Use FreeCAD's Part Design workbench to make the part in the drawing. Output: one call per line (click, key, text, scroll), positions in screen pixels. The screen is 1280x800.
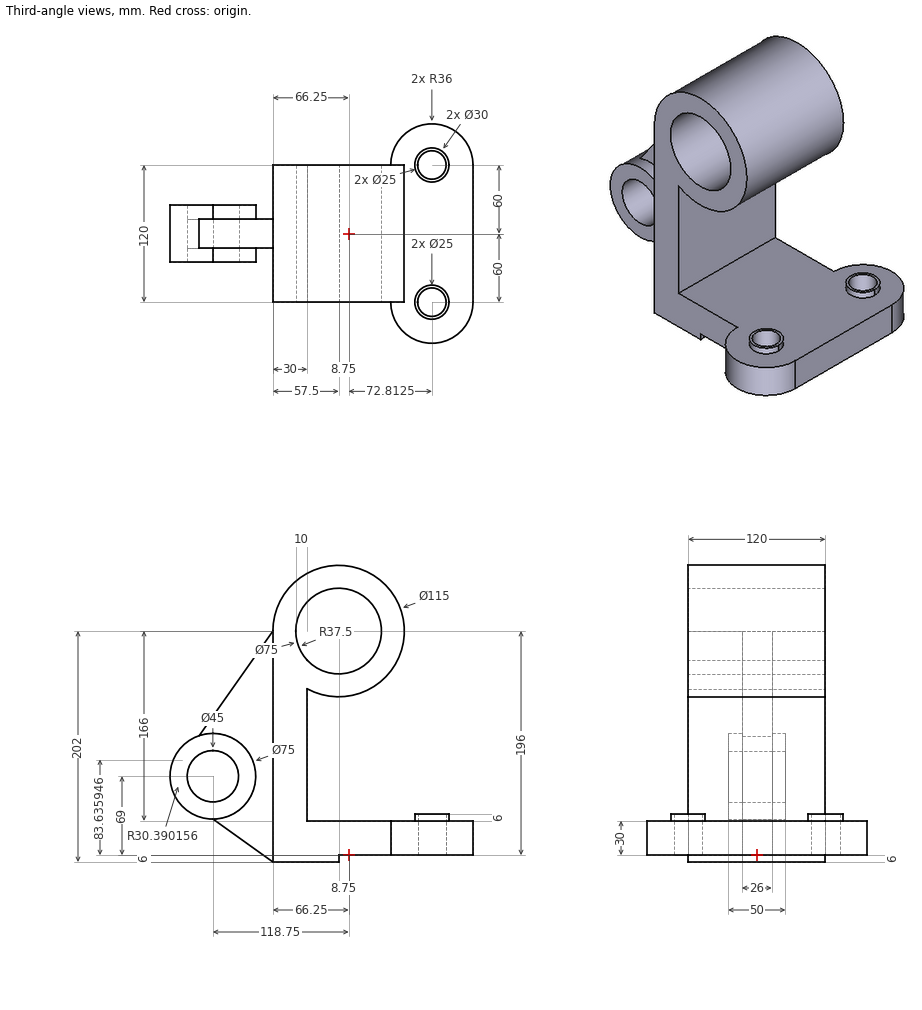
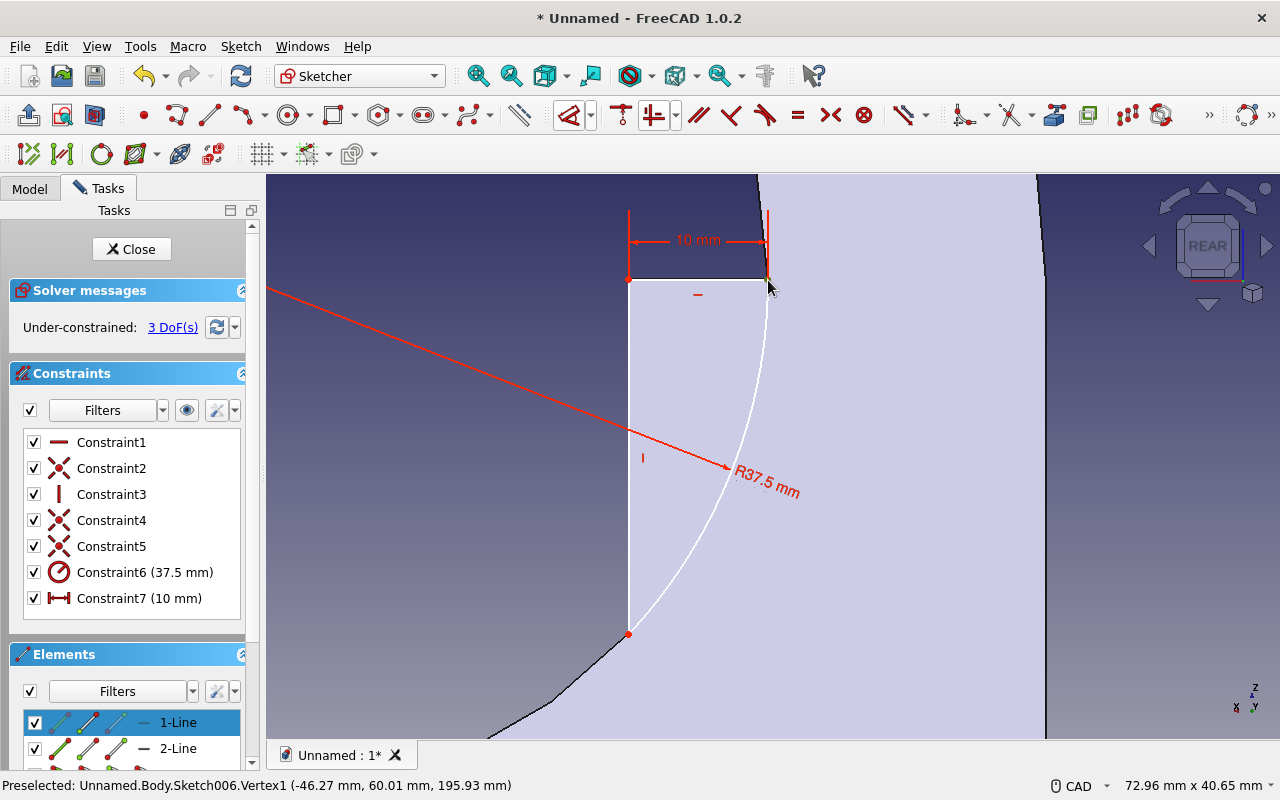
key(i)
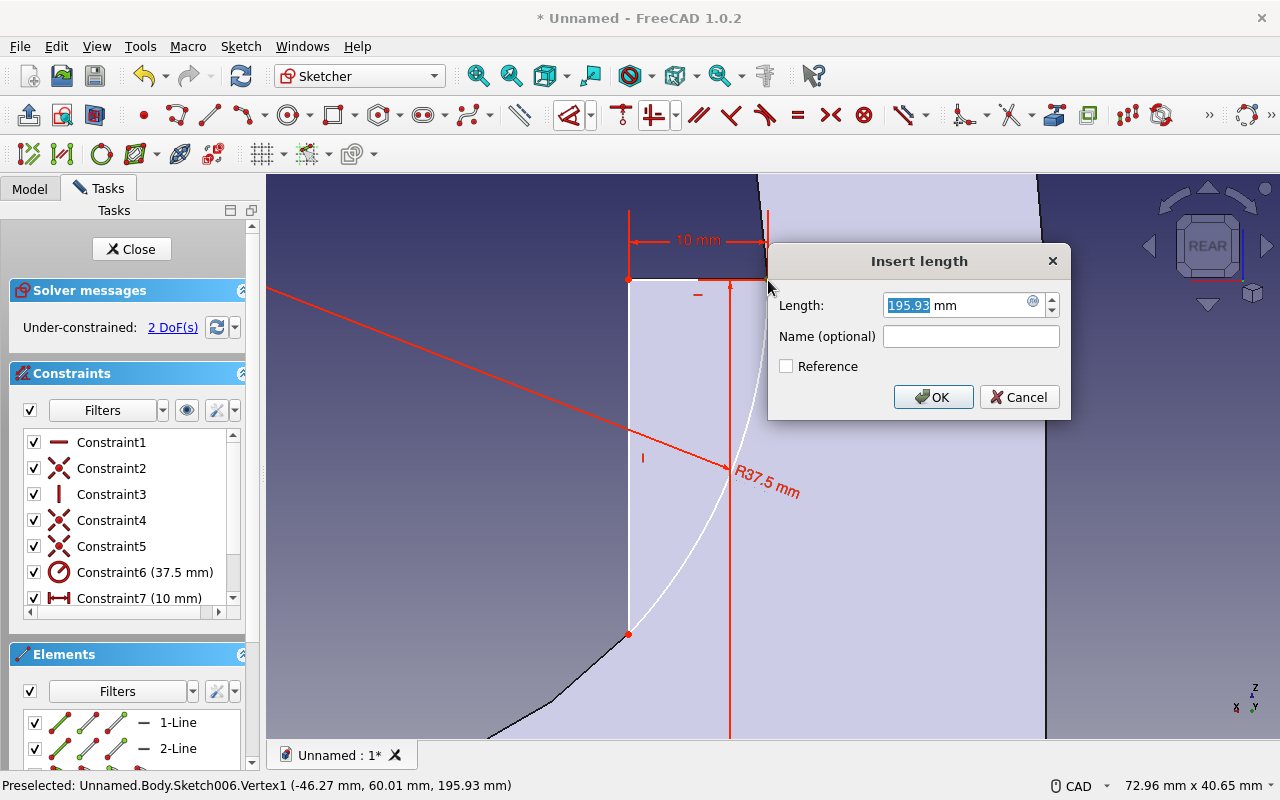
text(196)
key(Return)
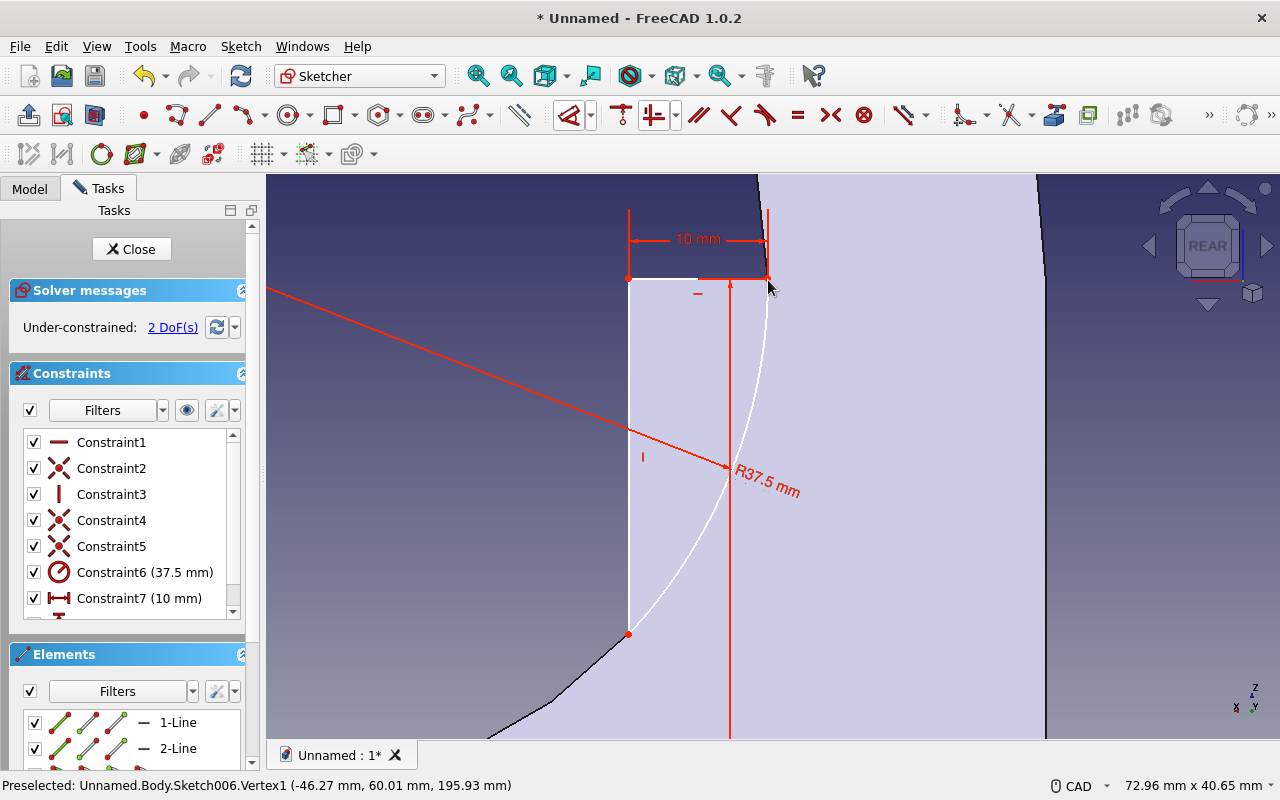
scroll(1115, 458, down, 1)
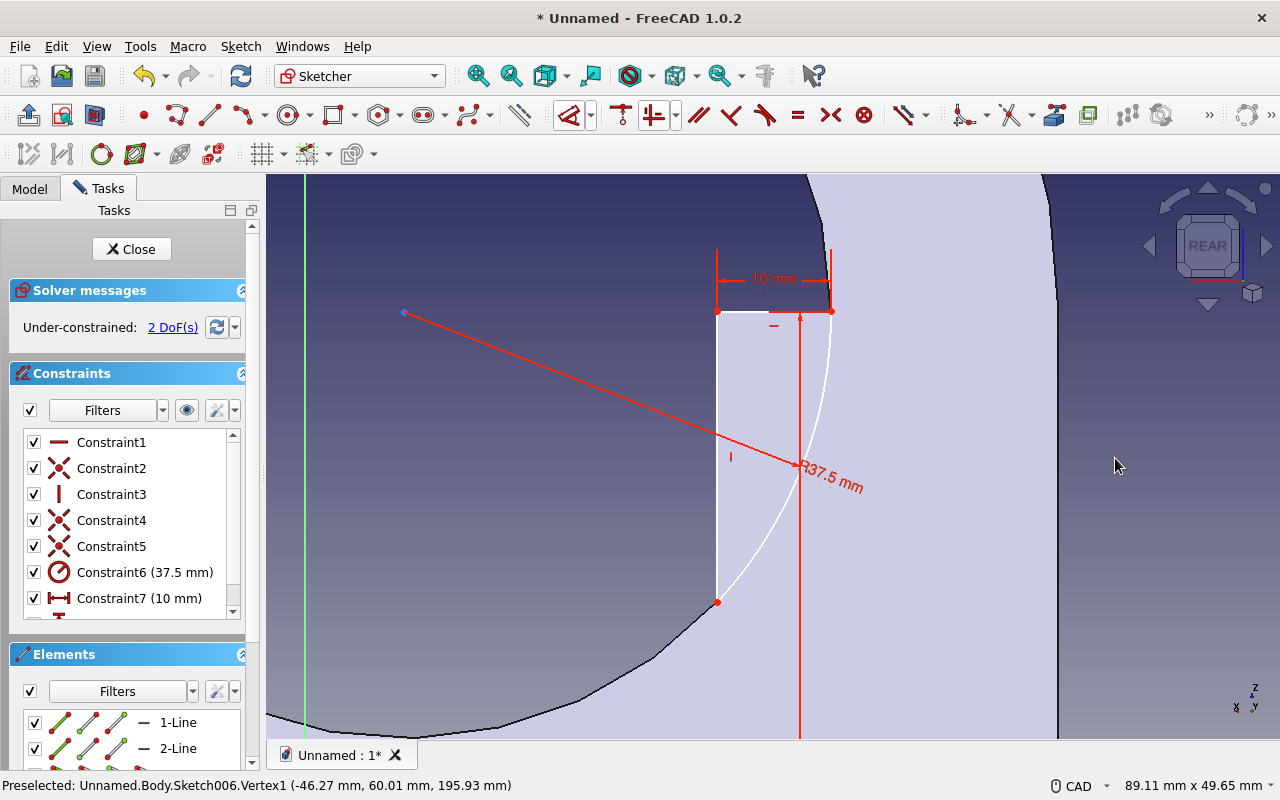
click(404, 312)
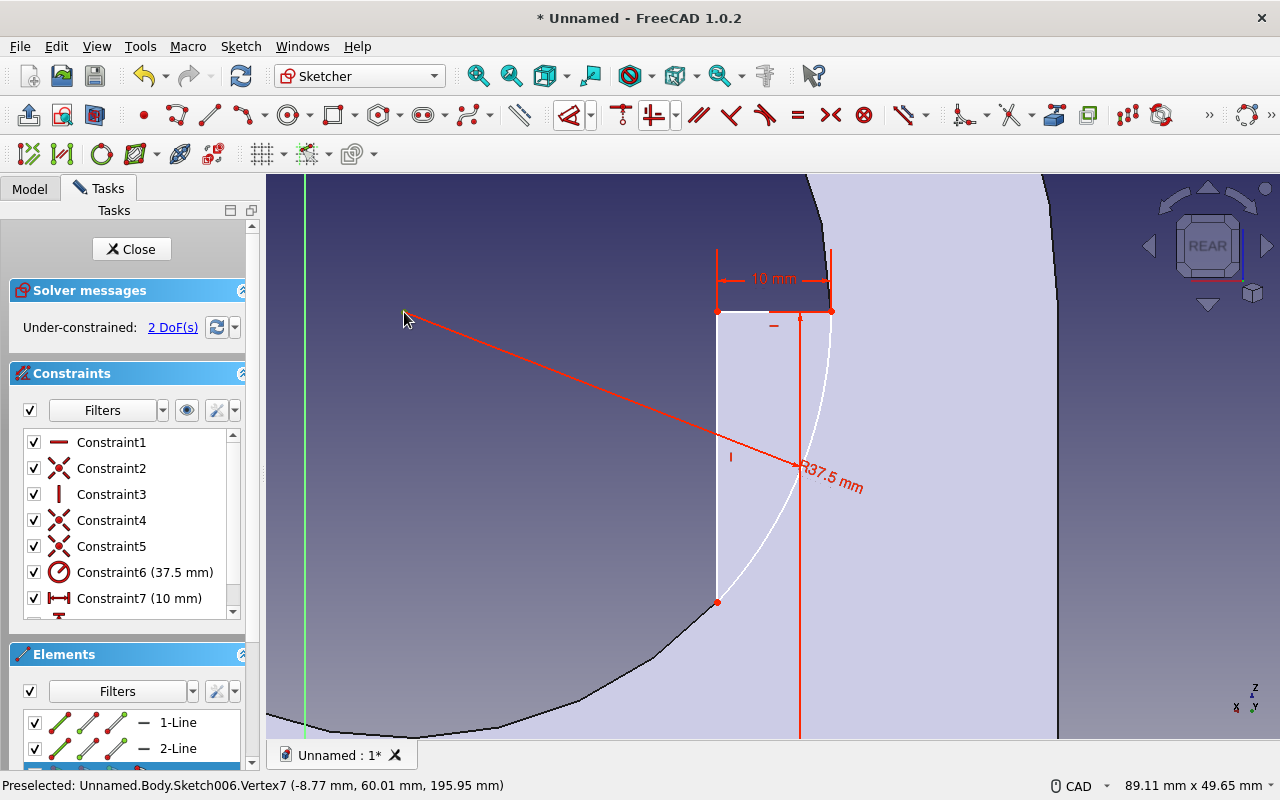
key(i)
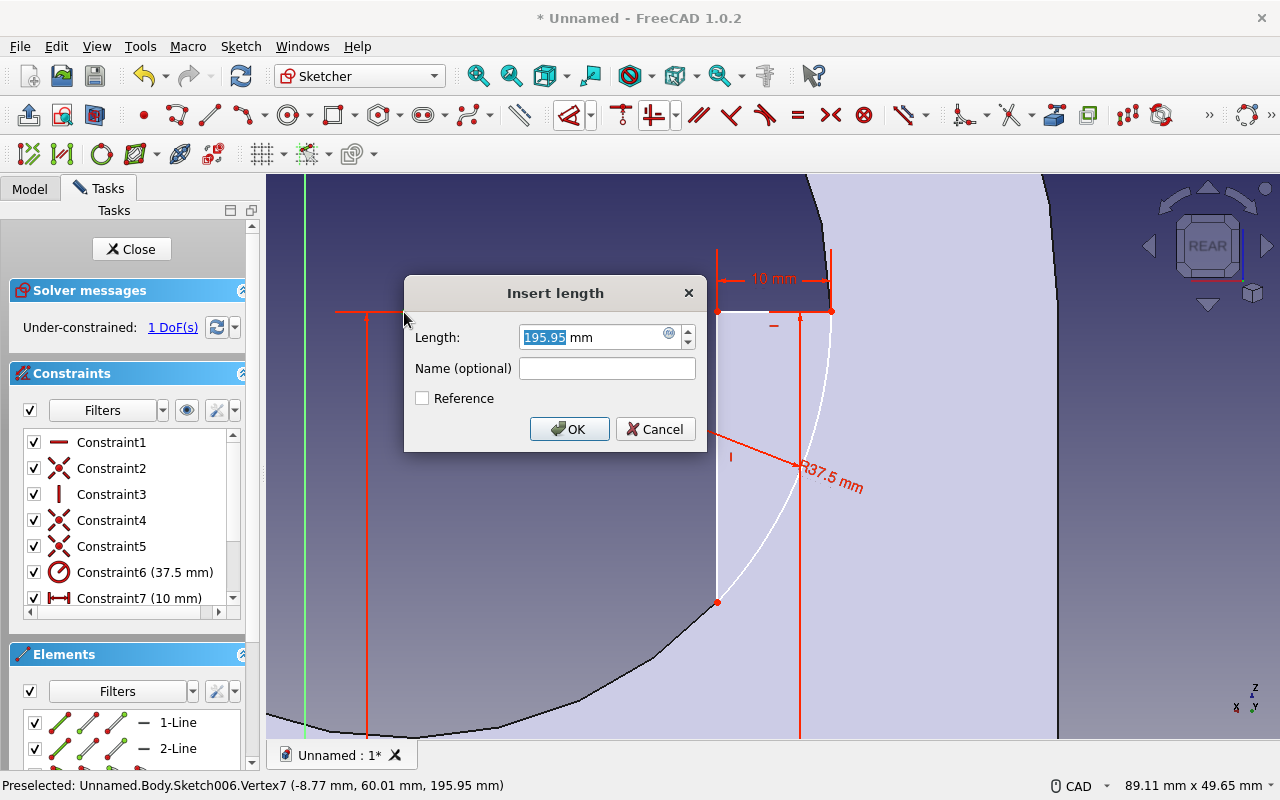
text(196)
key(Return)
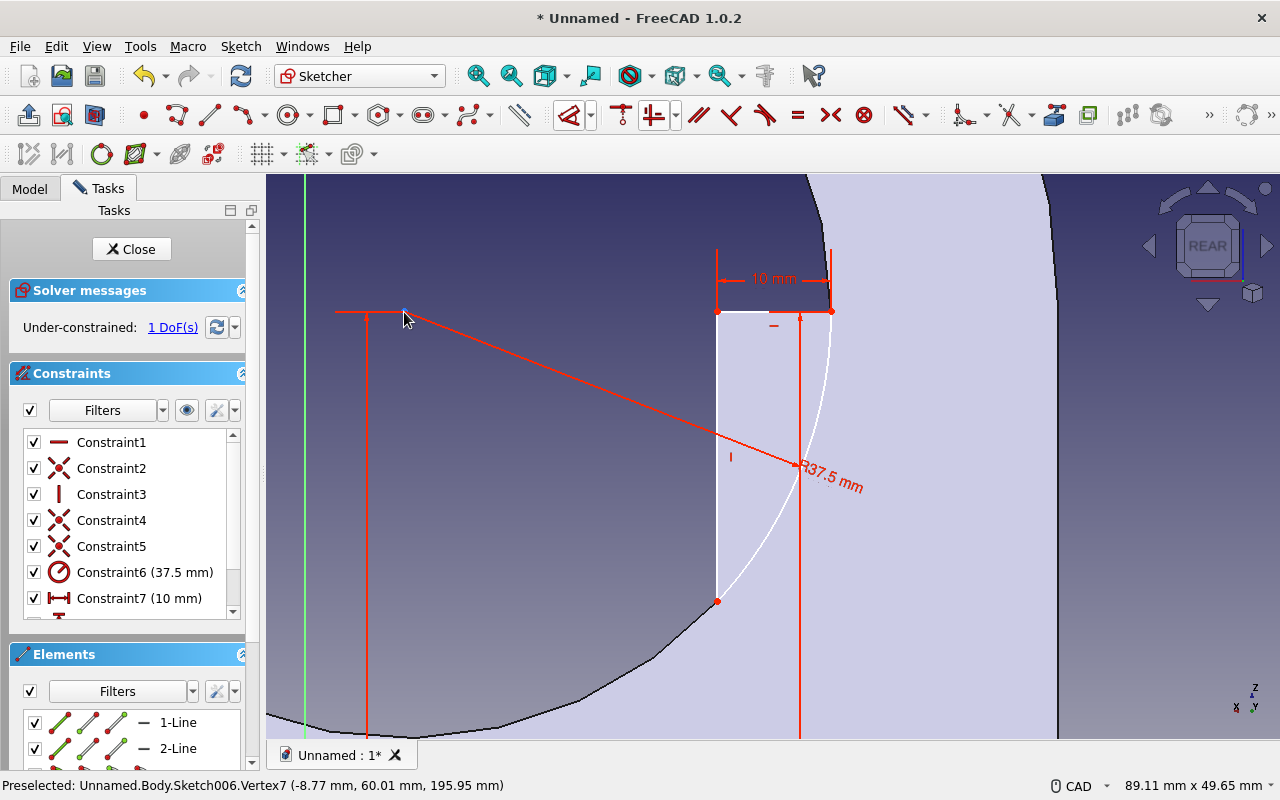
click(404, 312)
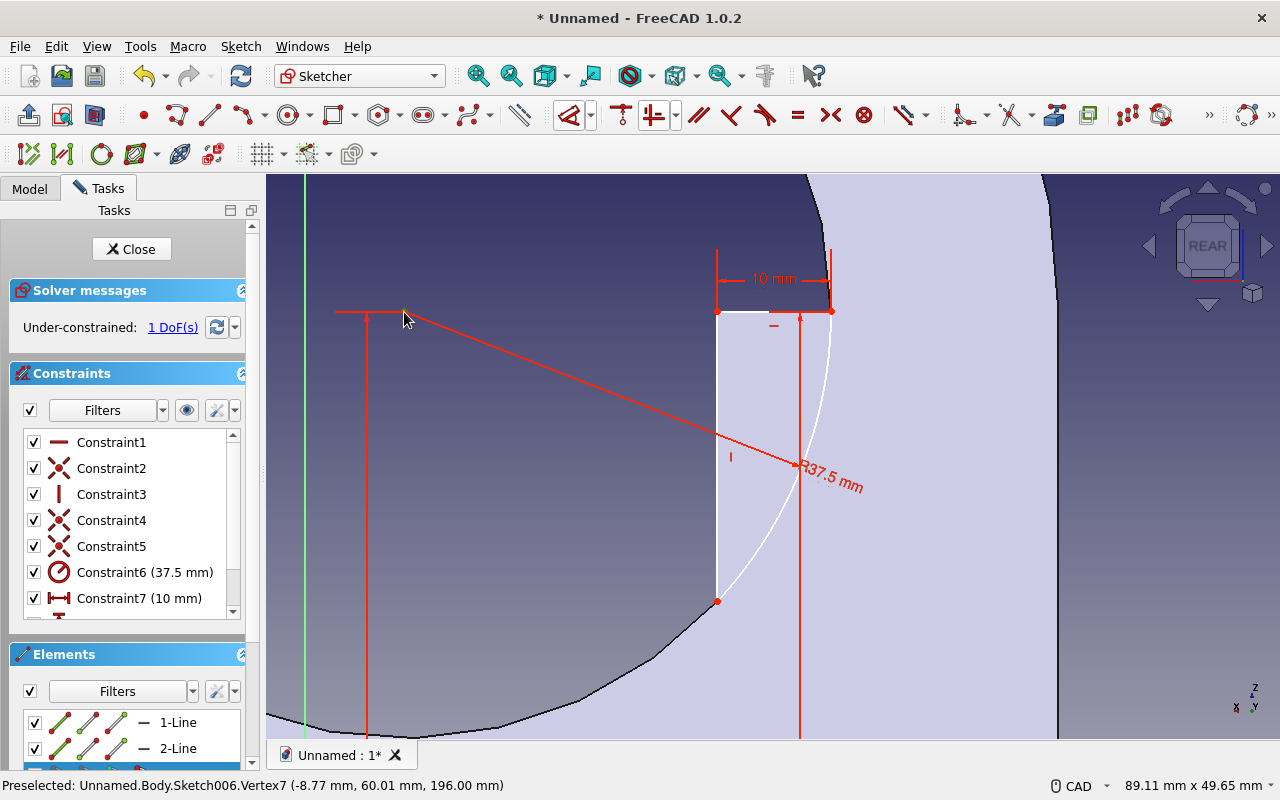
click(590, 116)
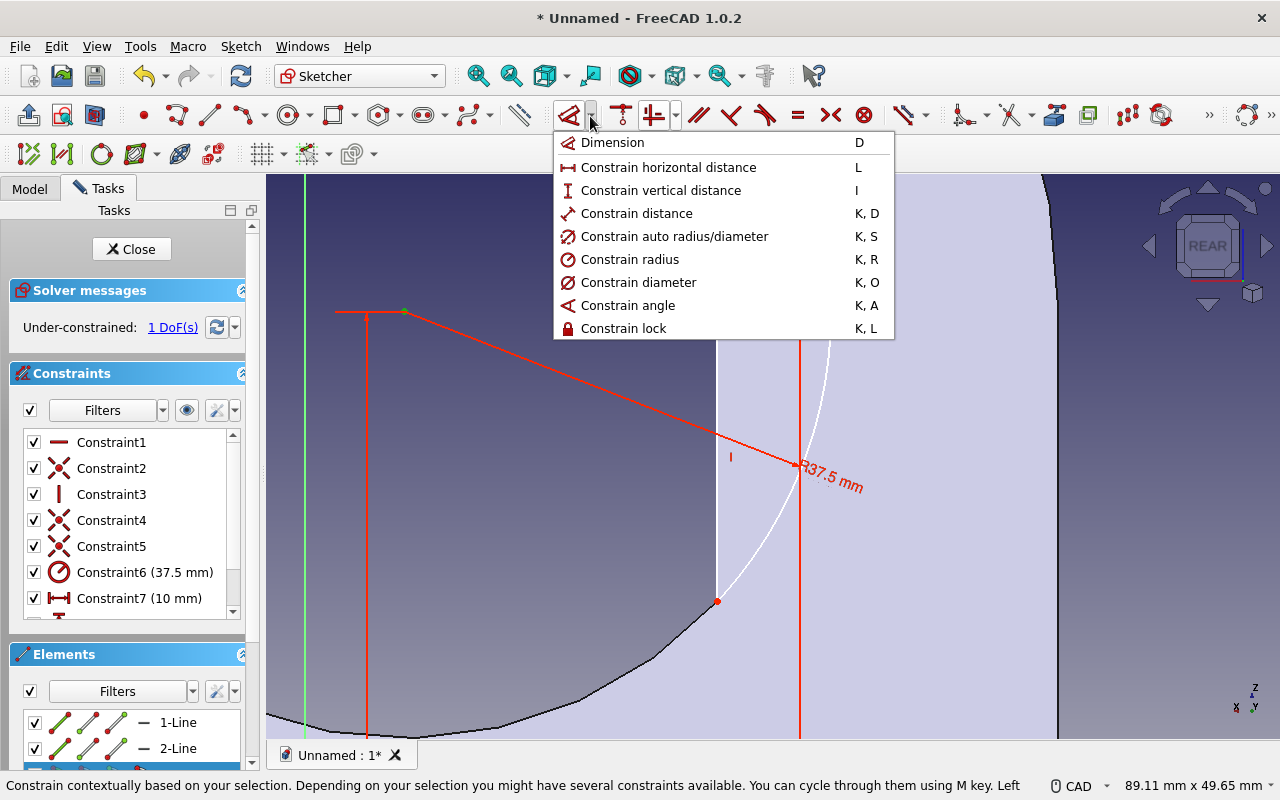
click(724, 168)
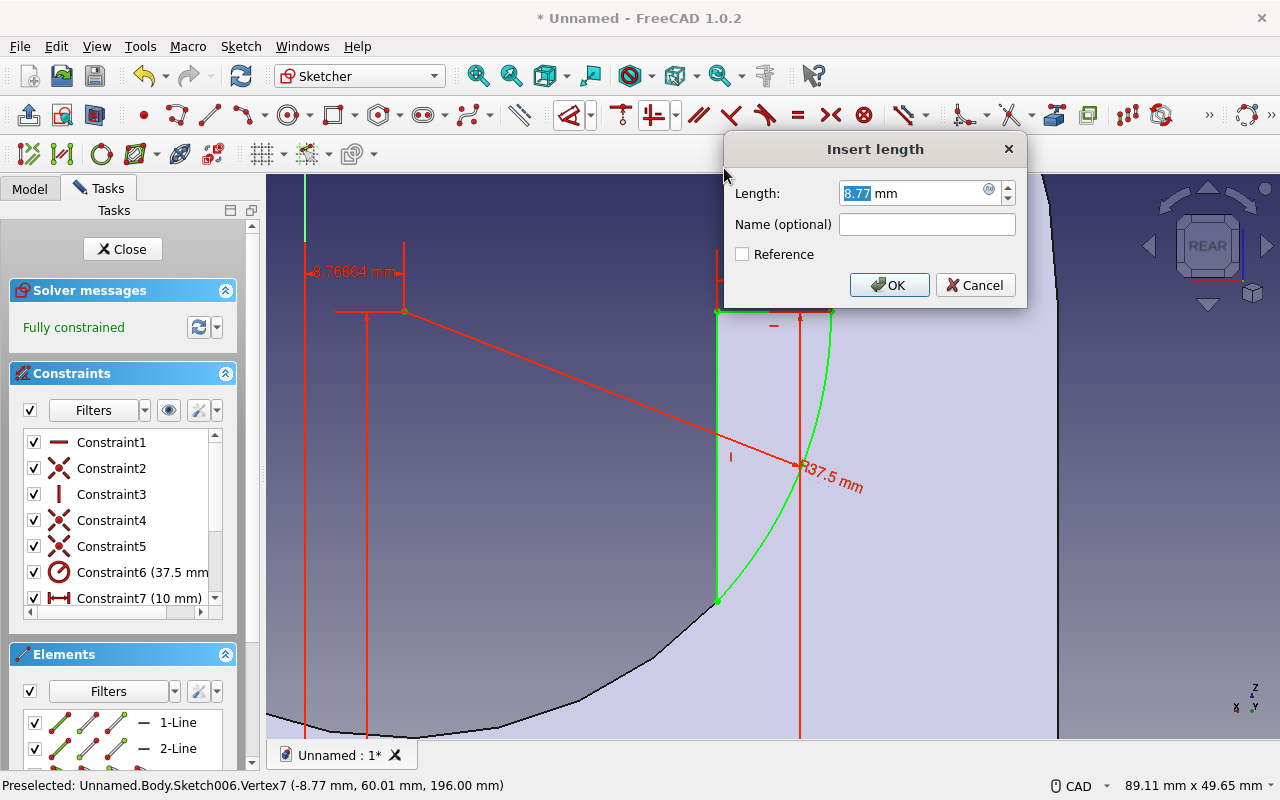
text(8.75)
key(Return)